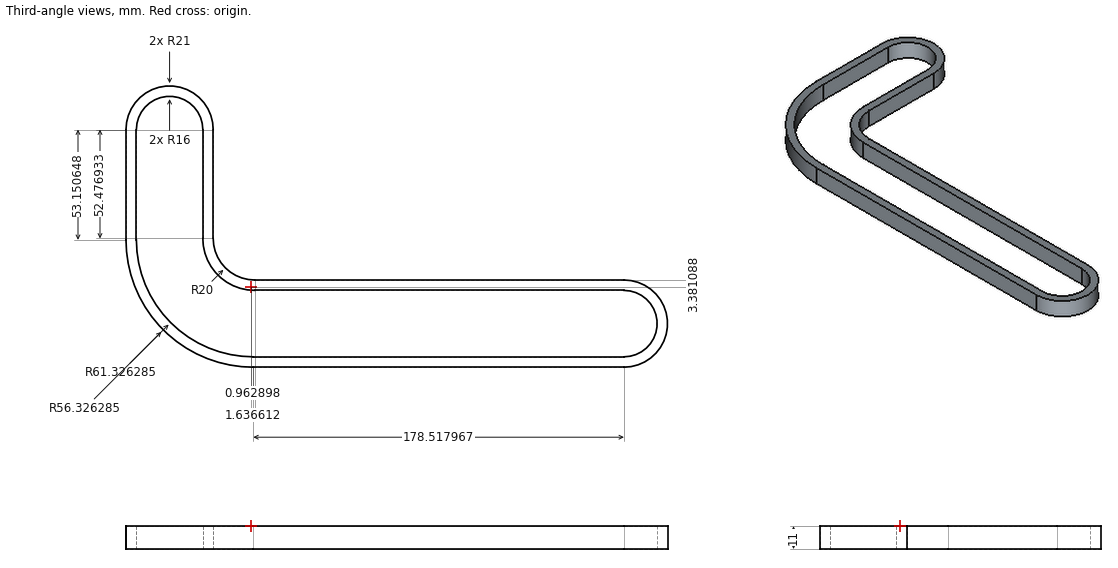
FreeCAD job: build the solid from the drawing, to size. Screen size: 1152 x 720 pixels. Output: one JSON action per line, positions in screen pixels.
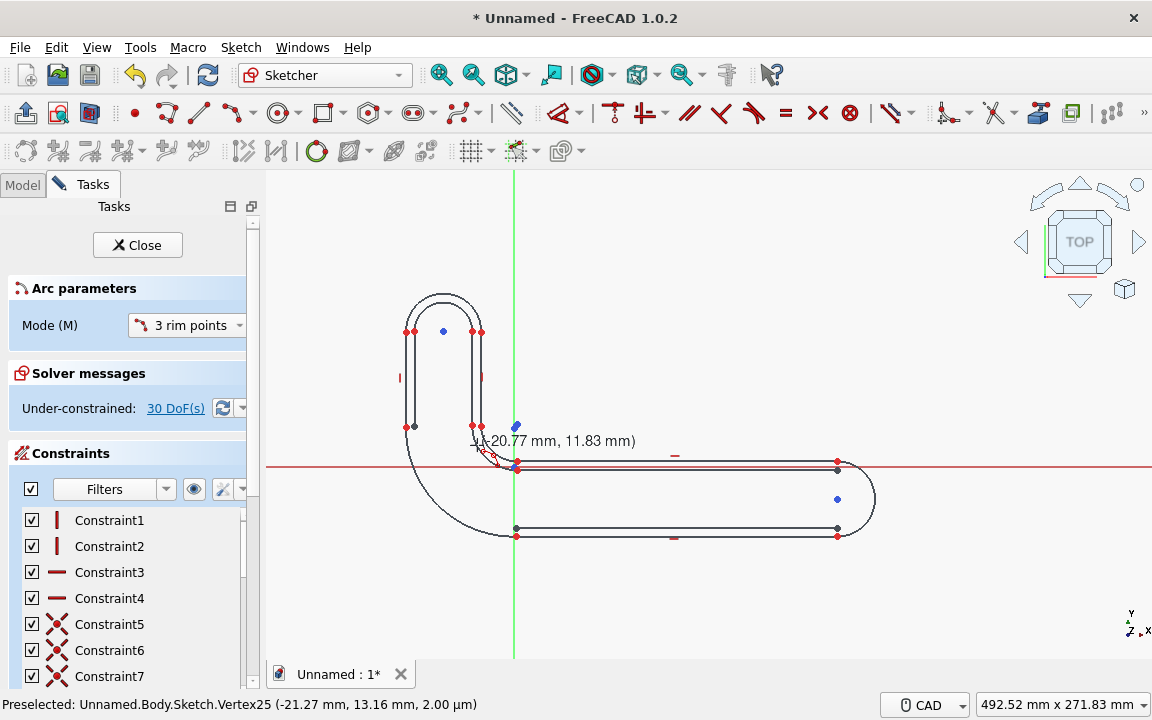
{"action": "scroll", "coordinate": [837, 470], "scroll_direction": "up", "scroll_amount": 9}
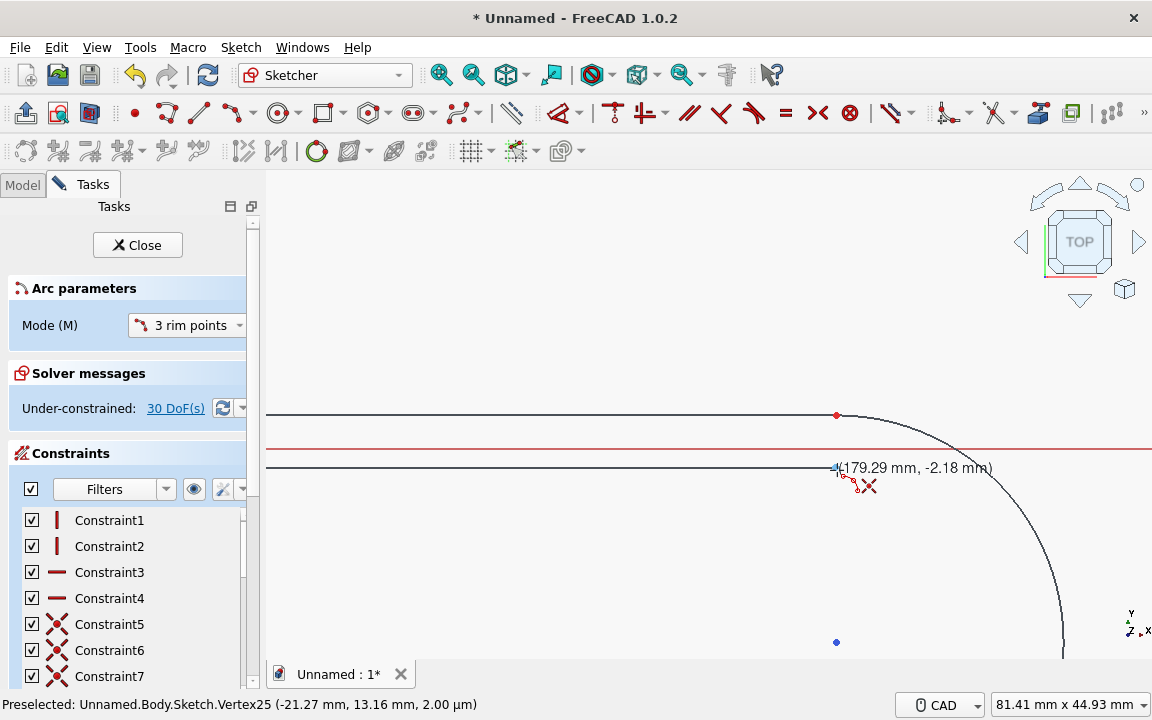
{"action": "left_click", "coordinate": [836, 468]}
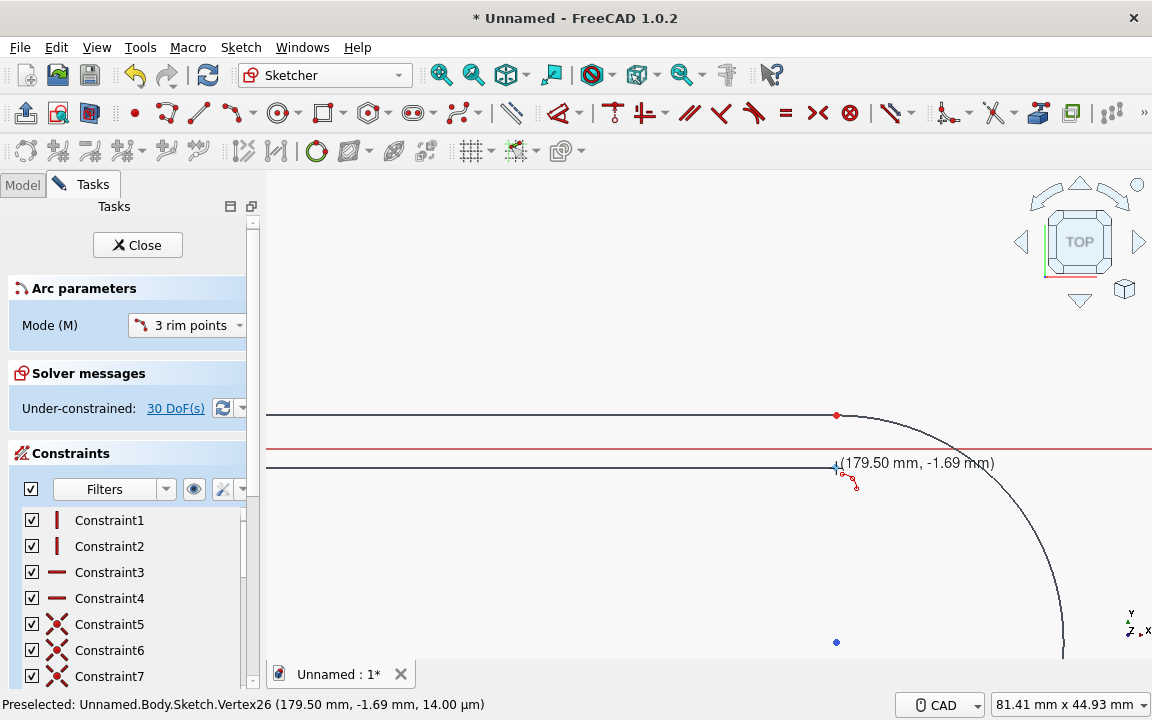
{"action": "scroll", "coordinate": [838, 470], "scroll_direction": "down", "scroll_amount": 9}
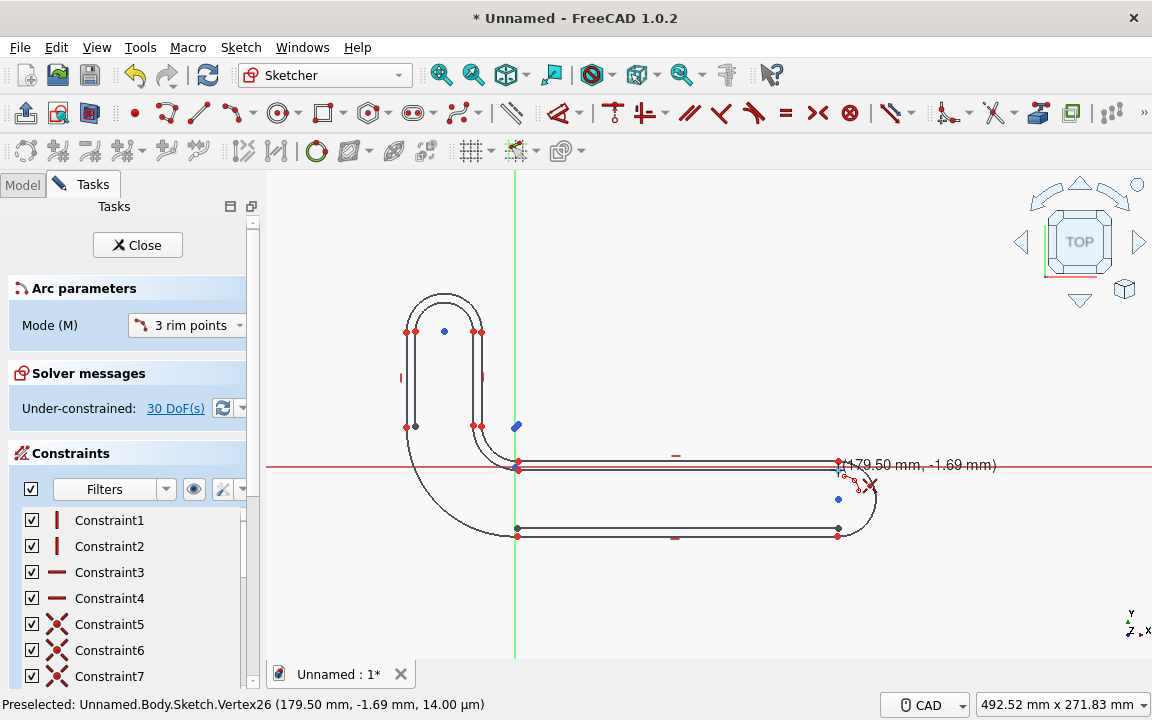
{"action": "scroll", "coordinate": [838, 528], "scroll_direction": "up", "scroll_amount": 3}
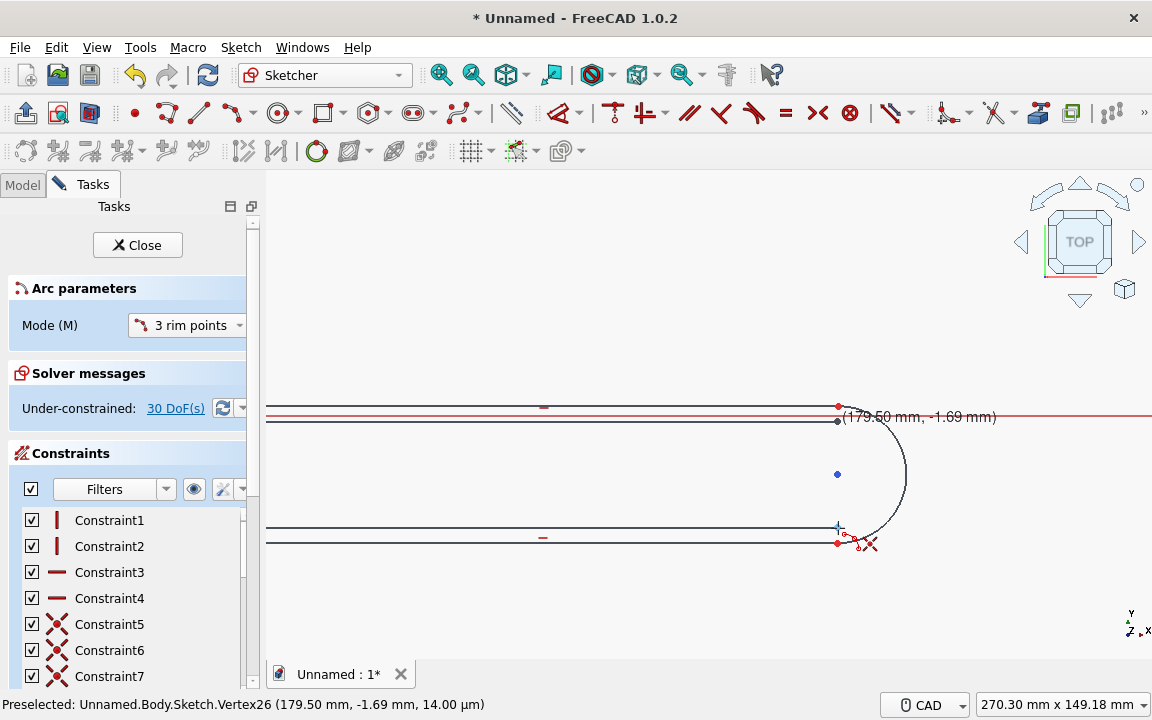
{"action": "left_click", "coordinate": [838, 528]}
{"action": "left_click", "coordinate": [880, 505]}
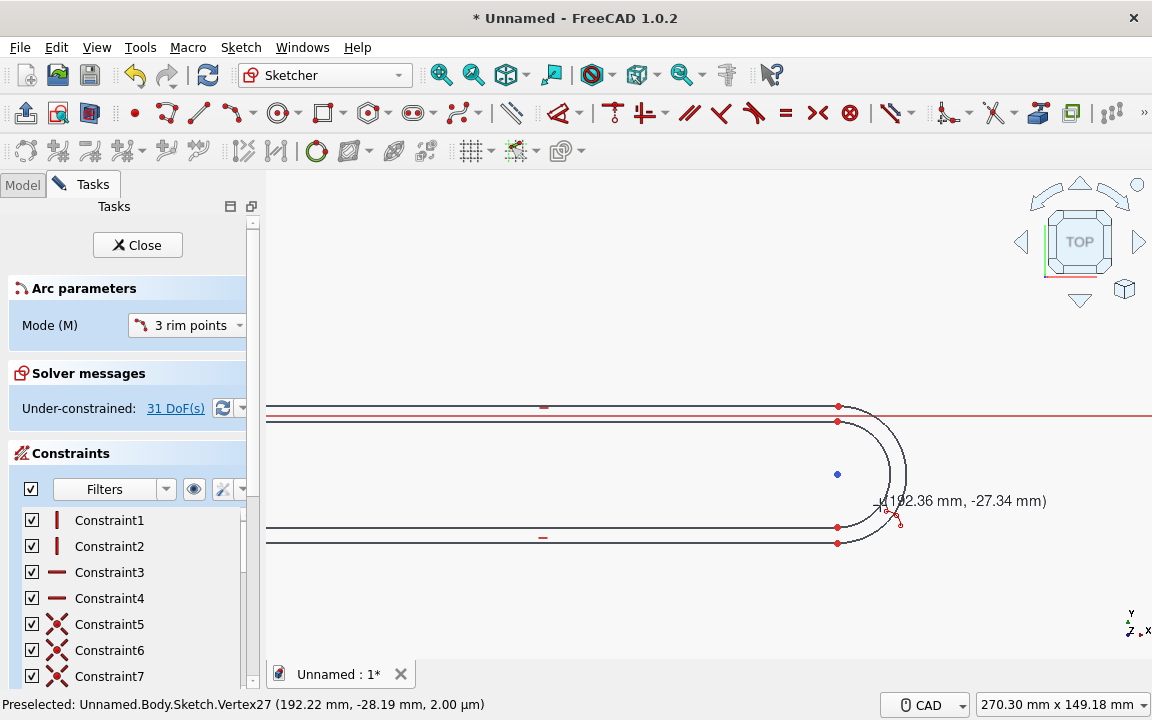
{"action": "scroll", "coordinate": [837, 528], "scroll_direction": "down", "scroll_amount": 3}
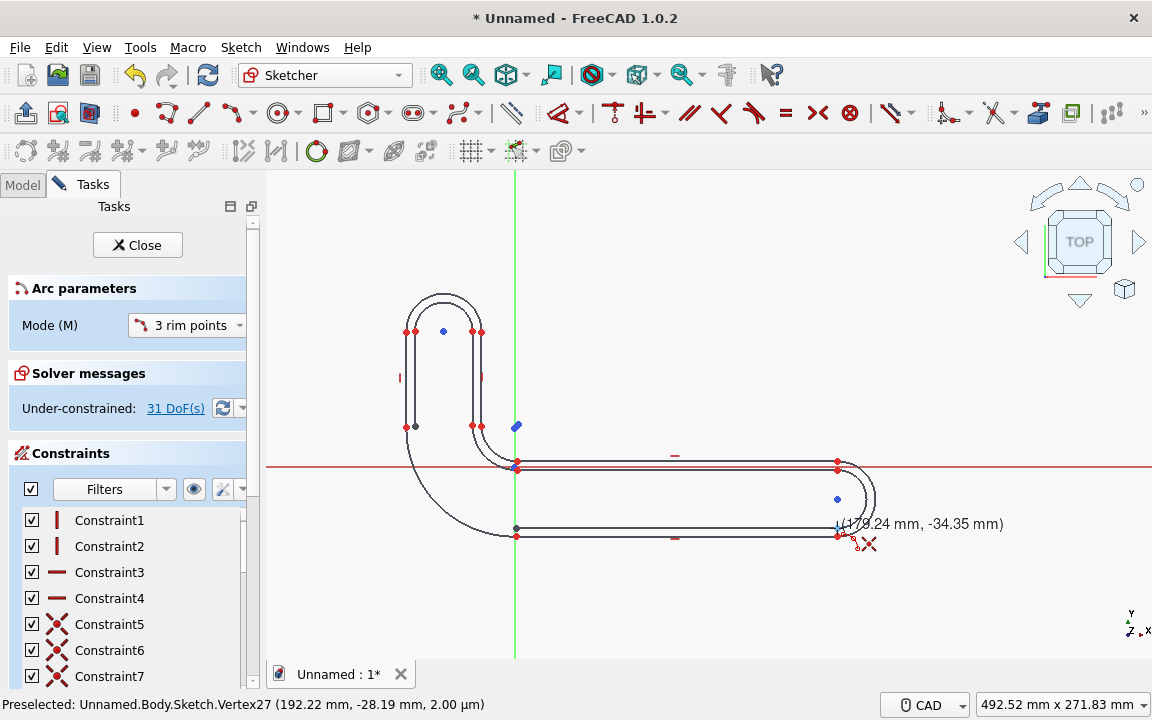
{"action": "scroll", "coordinate": [517, 528], "scroll_direction": "up", "scroll_amount": 12}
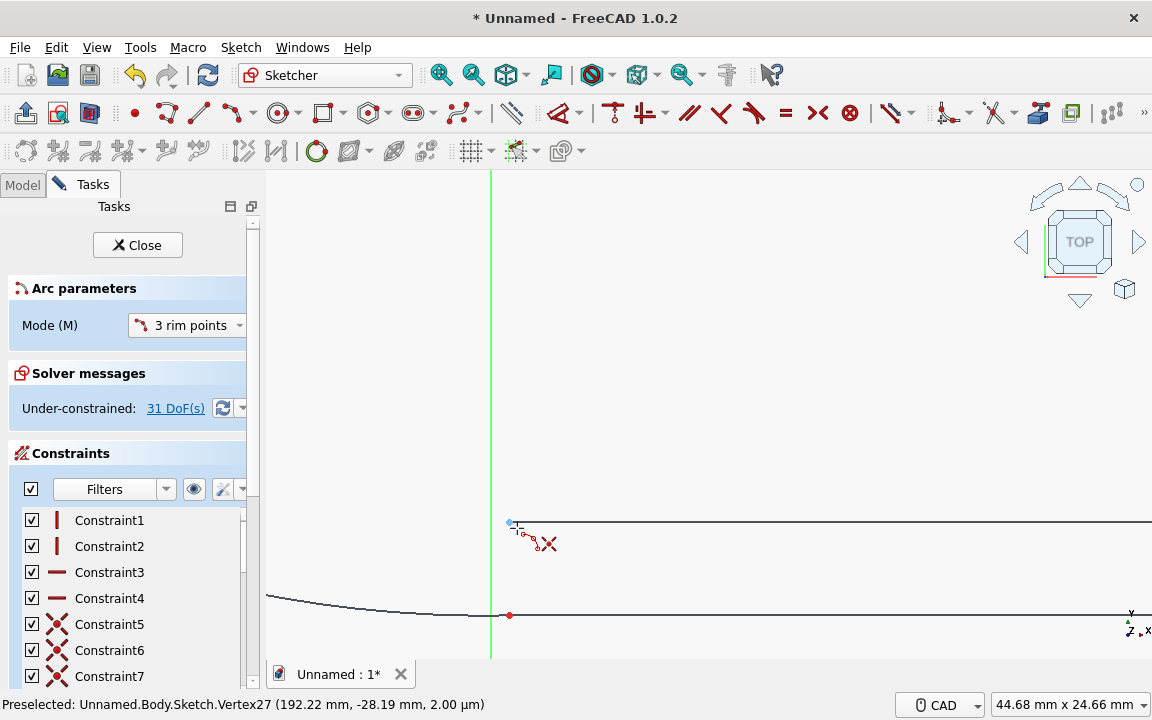
{"action": "left_click", "coordinate": [510, 522]}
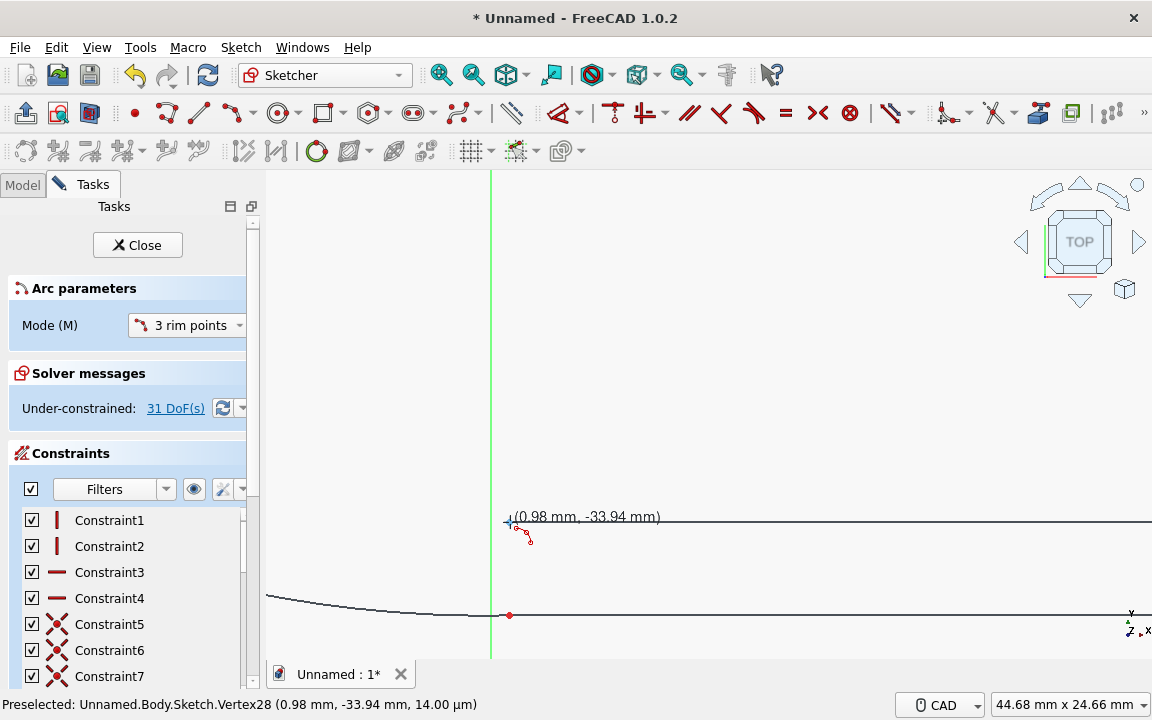
{"action": "scroll", "coordinate": [517, 529], "scroll_direction": "down", "scroll_amount": 12}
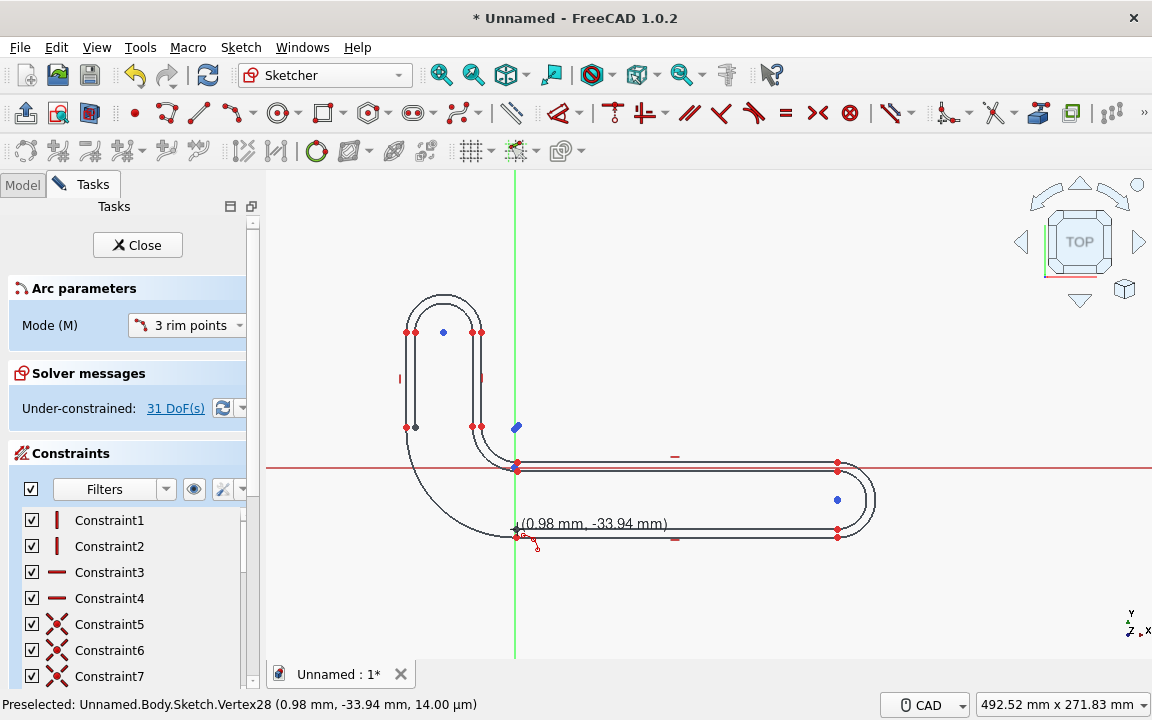
{"action": "scroll", "coordinate": [415, 427], "scroll_direction": "up", "scroll_amount": 3}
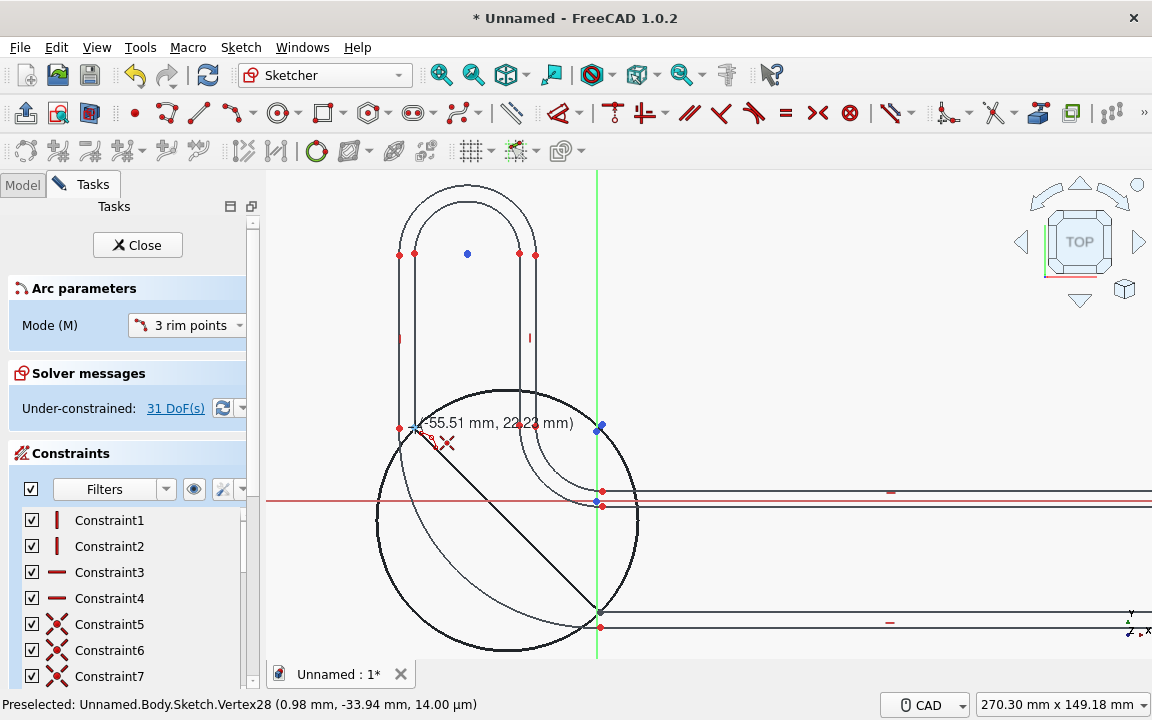
{"action": "left_click", "coordinate": [415, 428]}
{"action": "left_click", "coordinate": [469, 557]}
{"action": "key", "text": "Escape"}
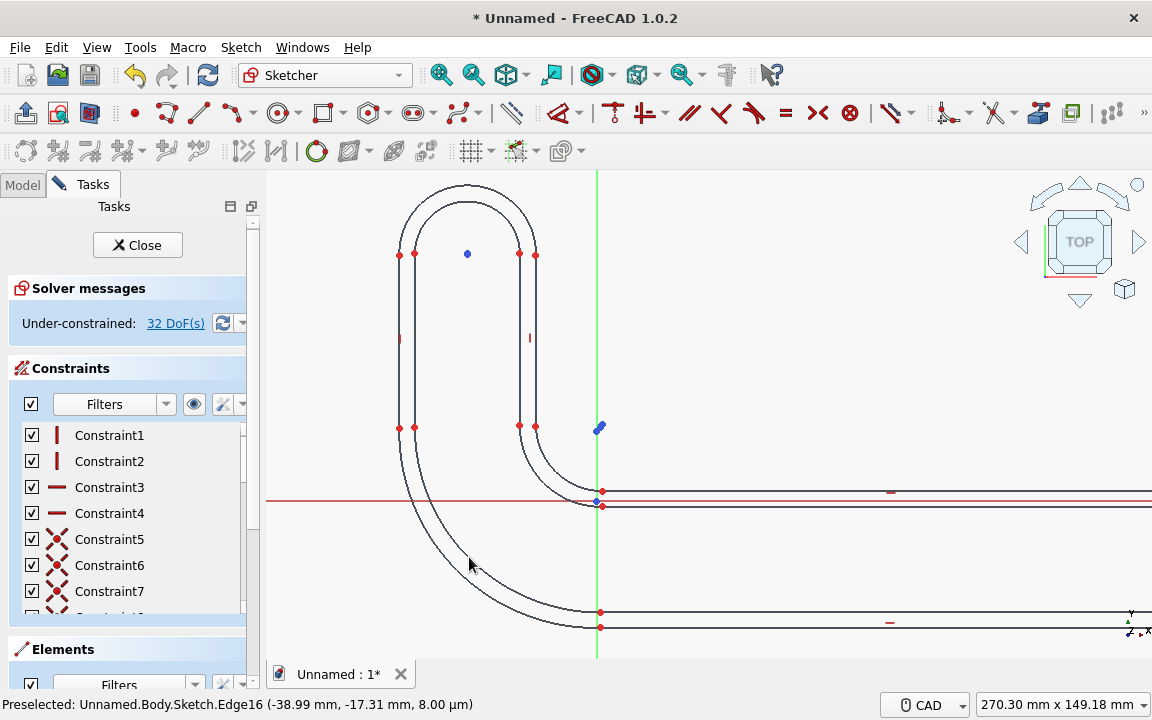
{"action": "left_click", "coordinate": [536, 375]}